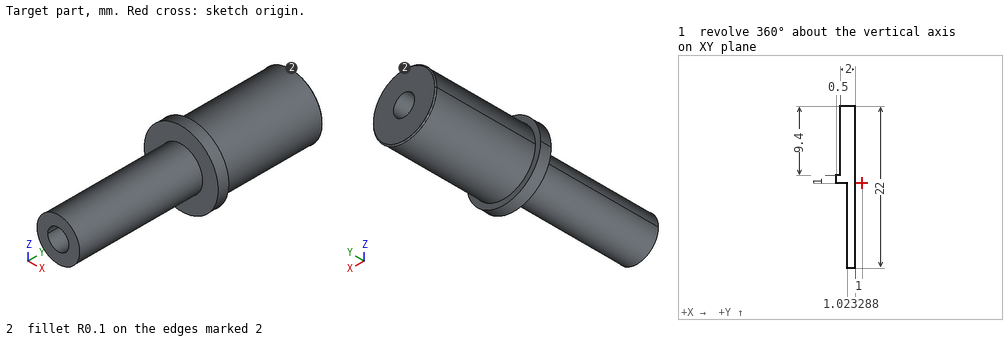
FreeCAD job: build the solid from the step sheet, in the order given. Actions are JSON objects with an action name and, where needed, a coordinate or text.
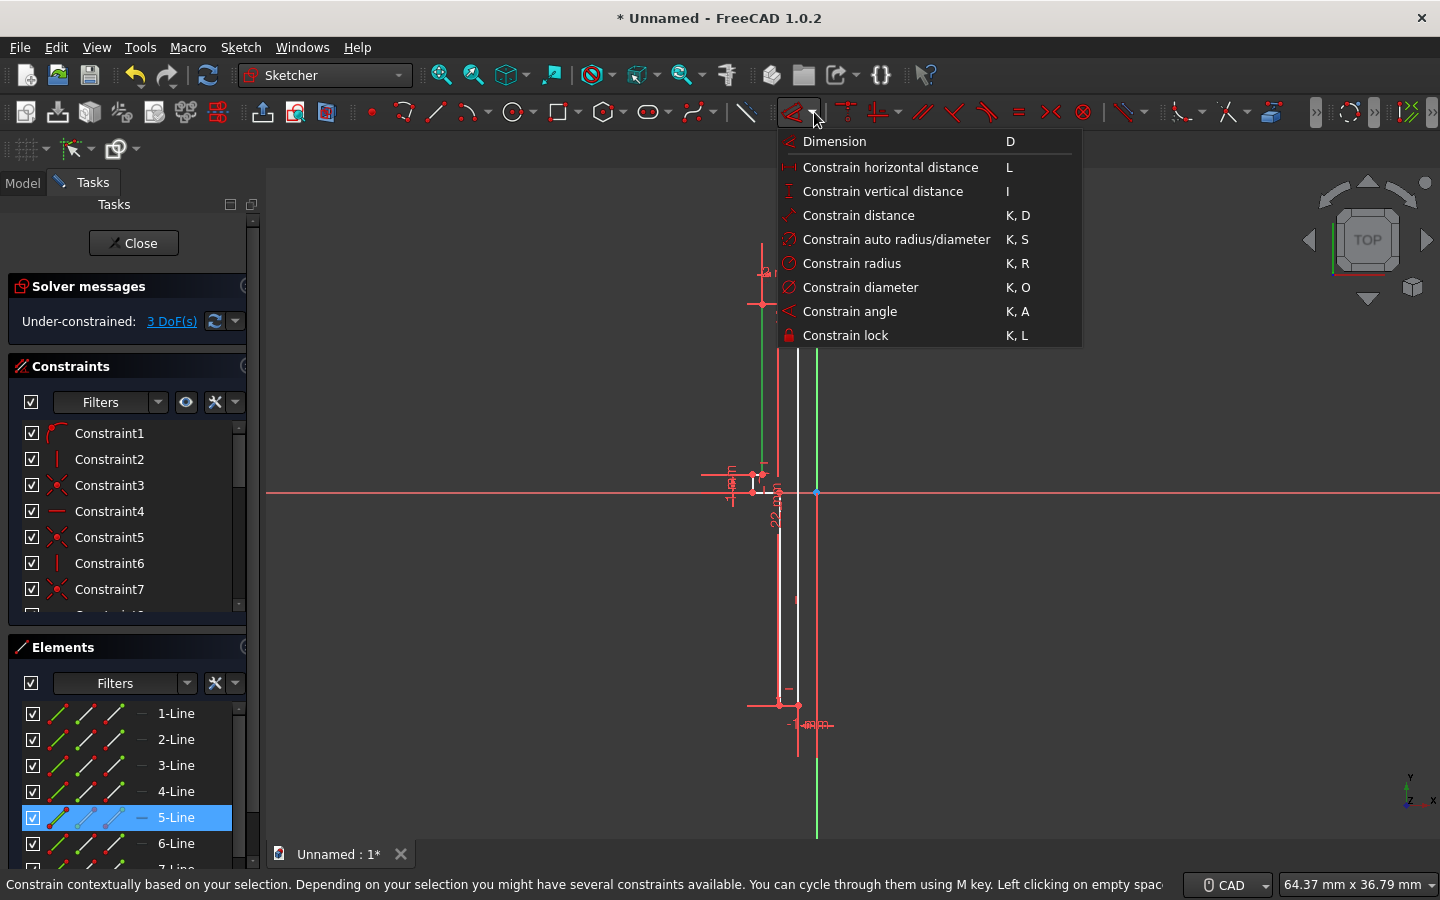
{"action": "left_click", "coordinate": [930, 191]}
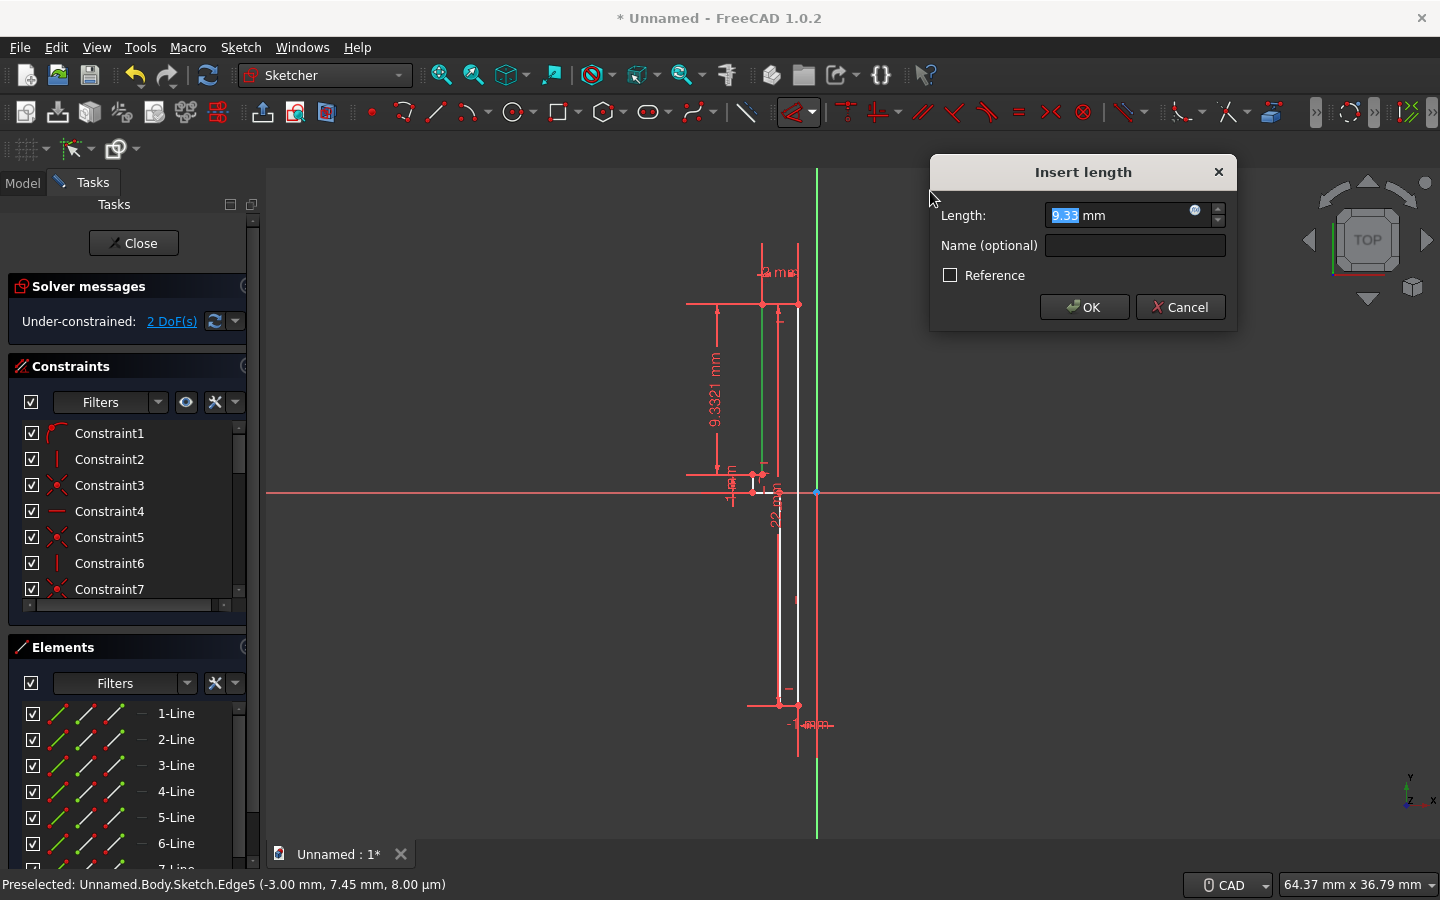
{"action": "type", "text": "9.4"}
{"action": "key", "text": "Return"}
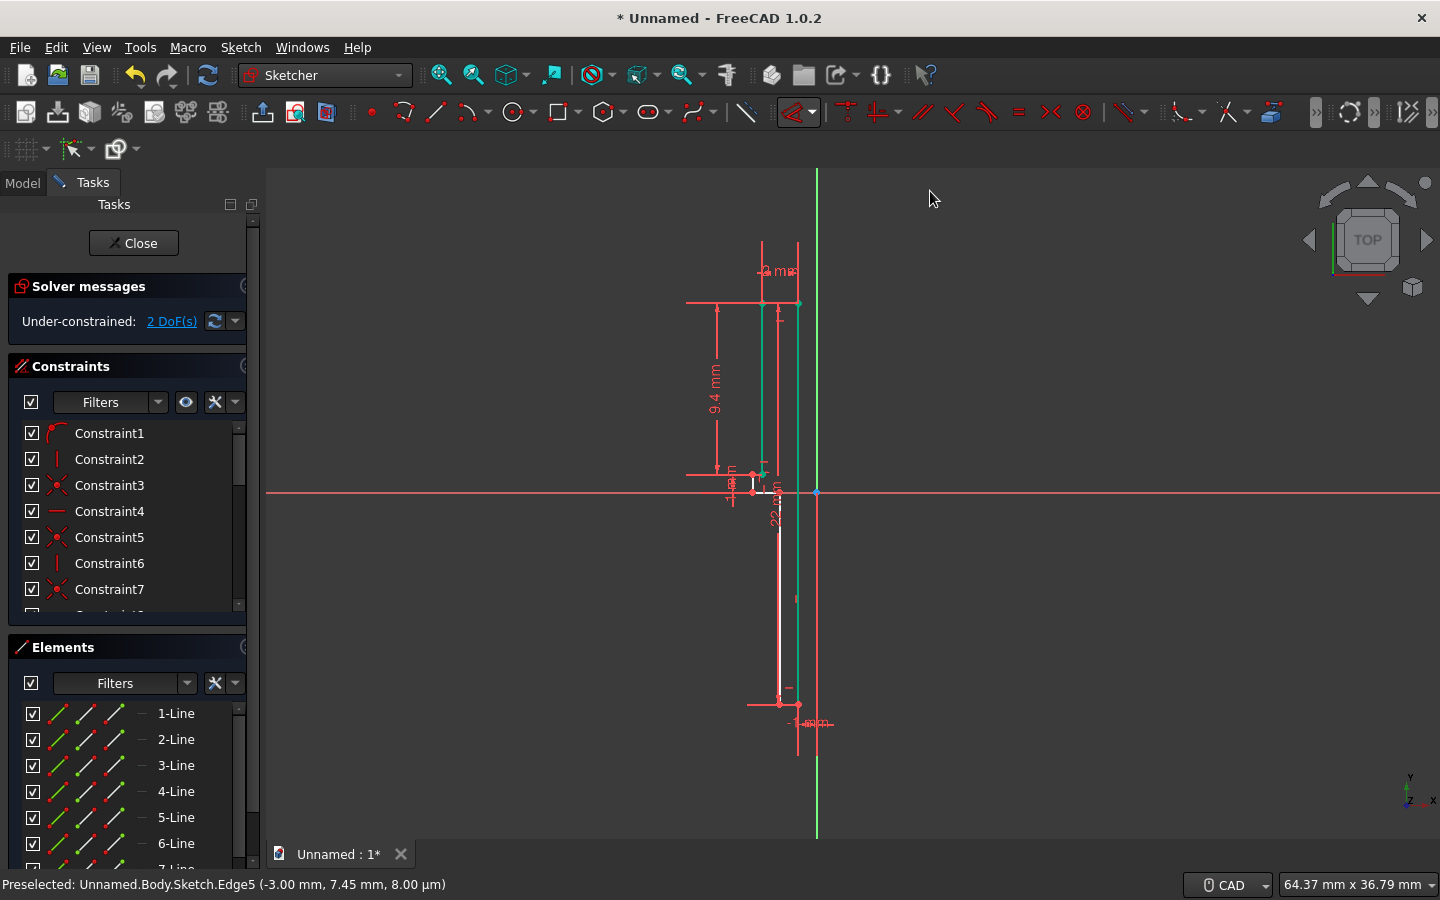
{"action": "scroll", "coordinate": [757, 475], "scroll_direction": "up", "scroll_amount": 8}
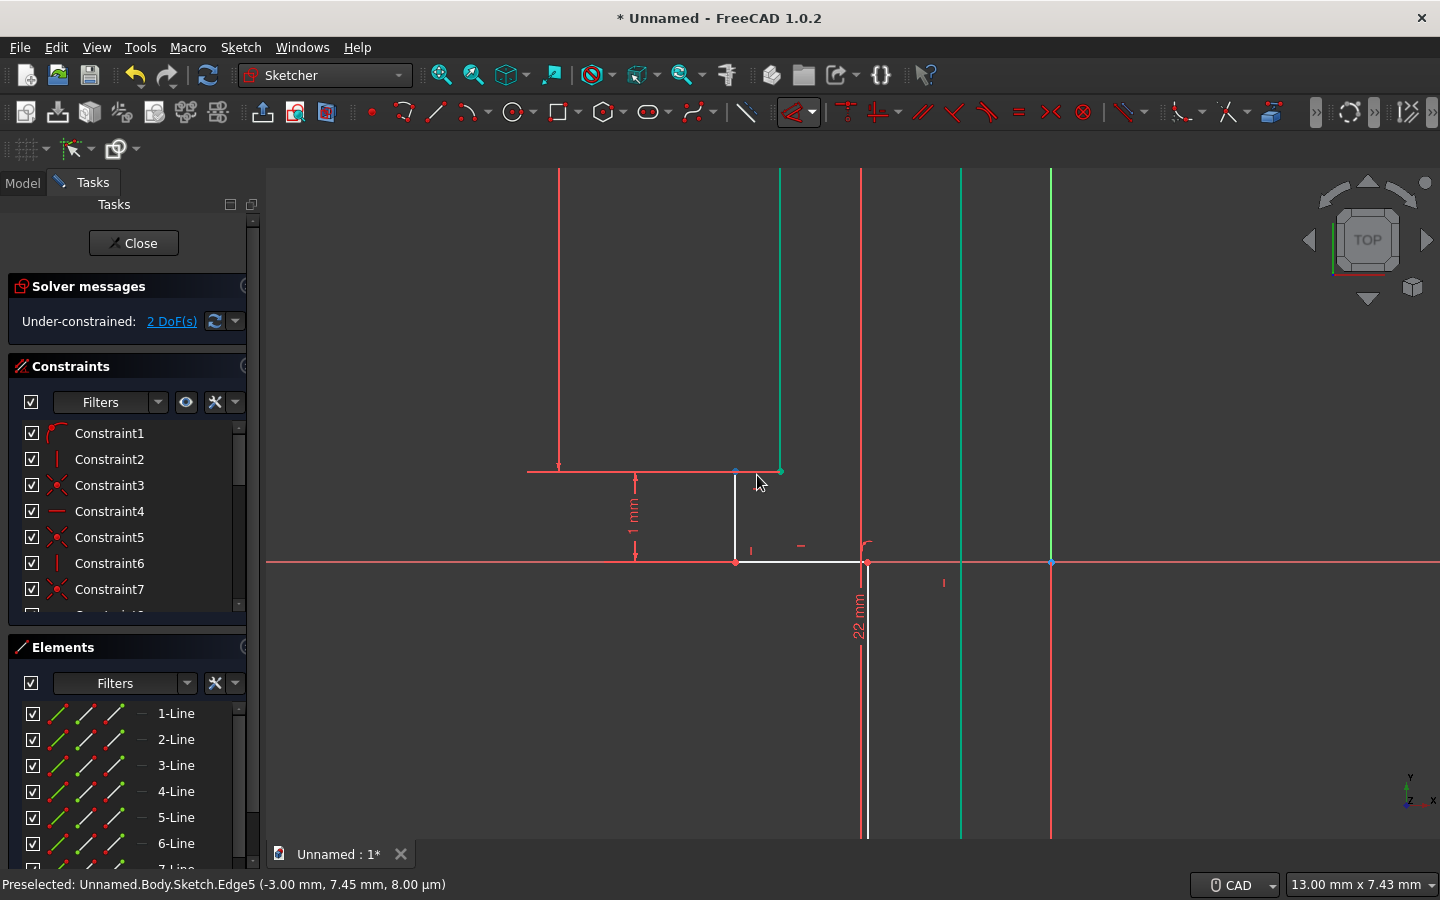
{"action": "left_click", "coordinate": [758, 472]}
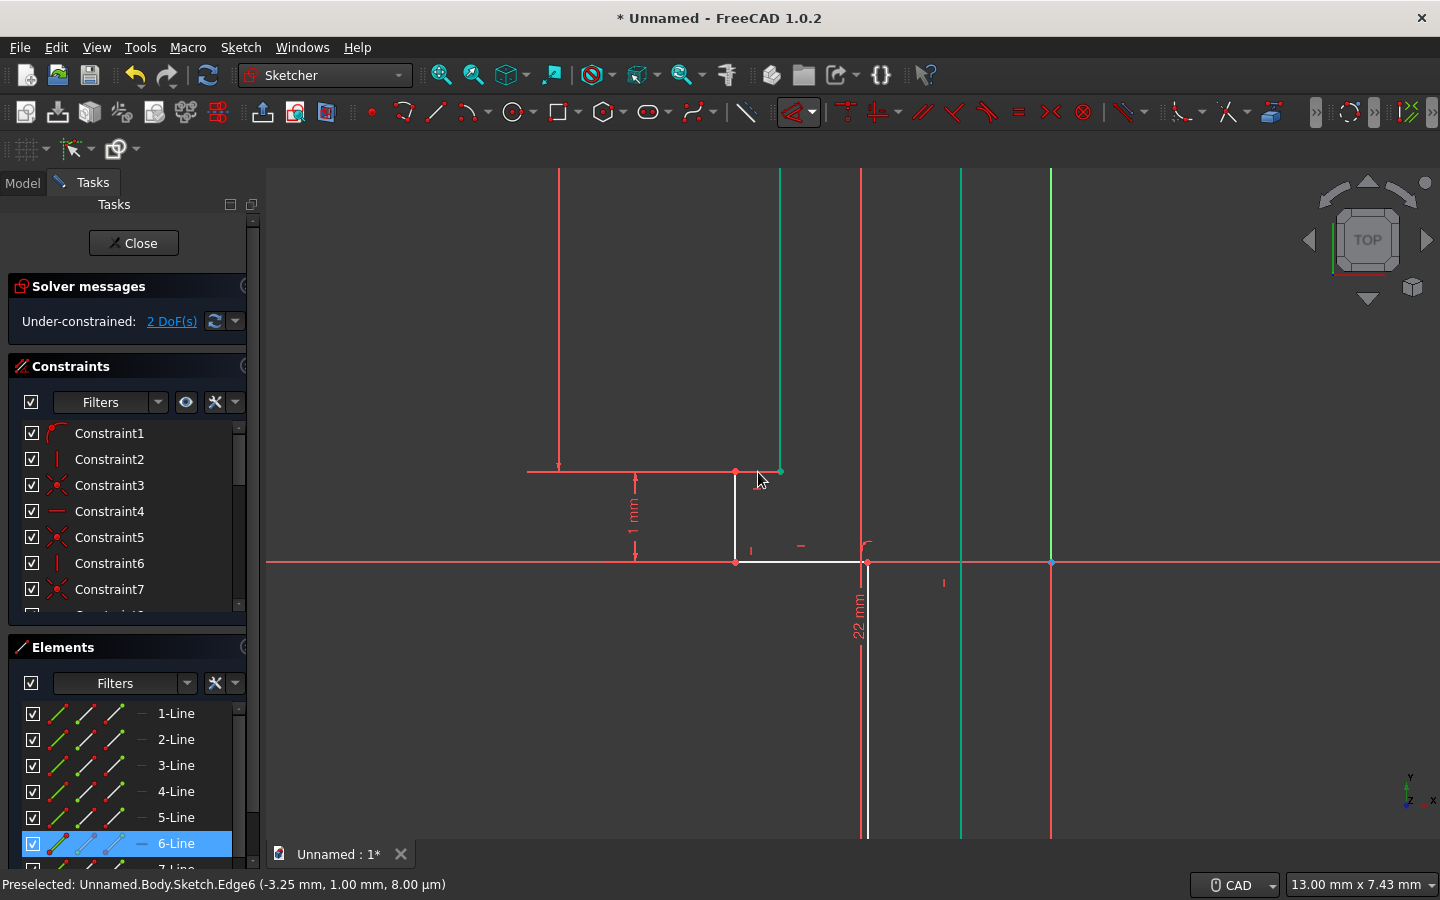
{"action": "left_click", "coordinate": [814, 112]}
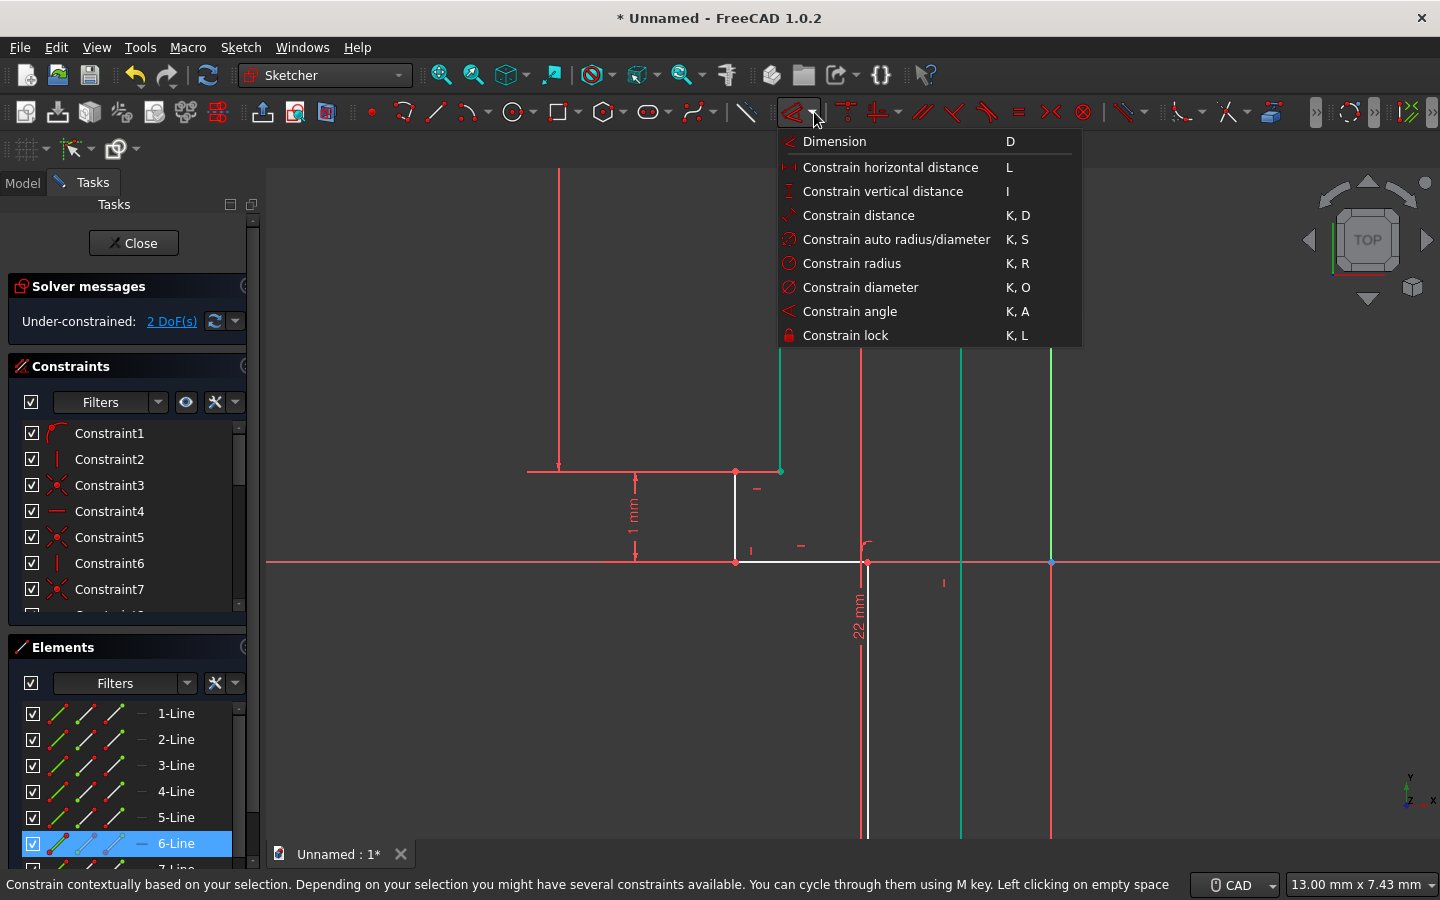
{"action": "left_click", "coordinate": [930, 167]}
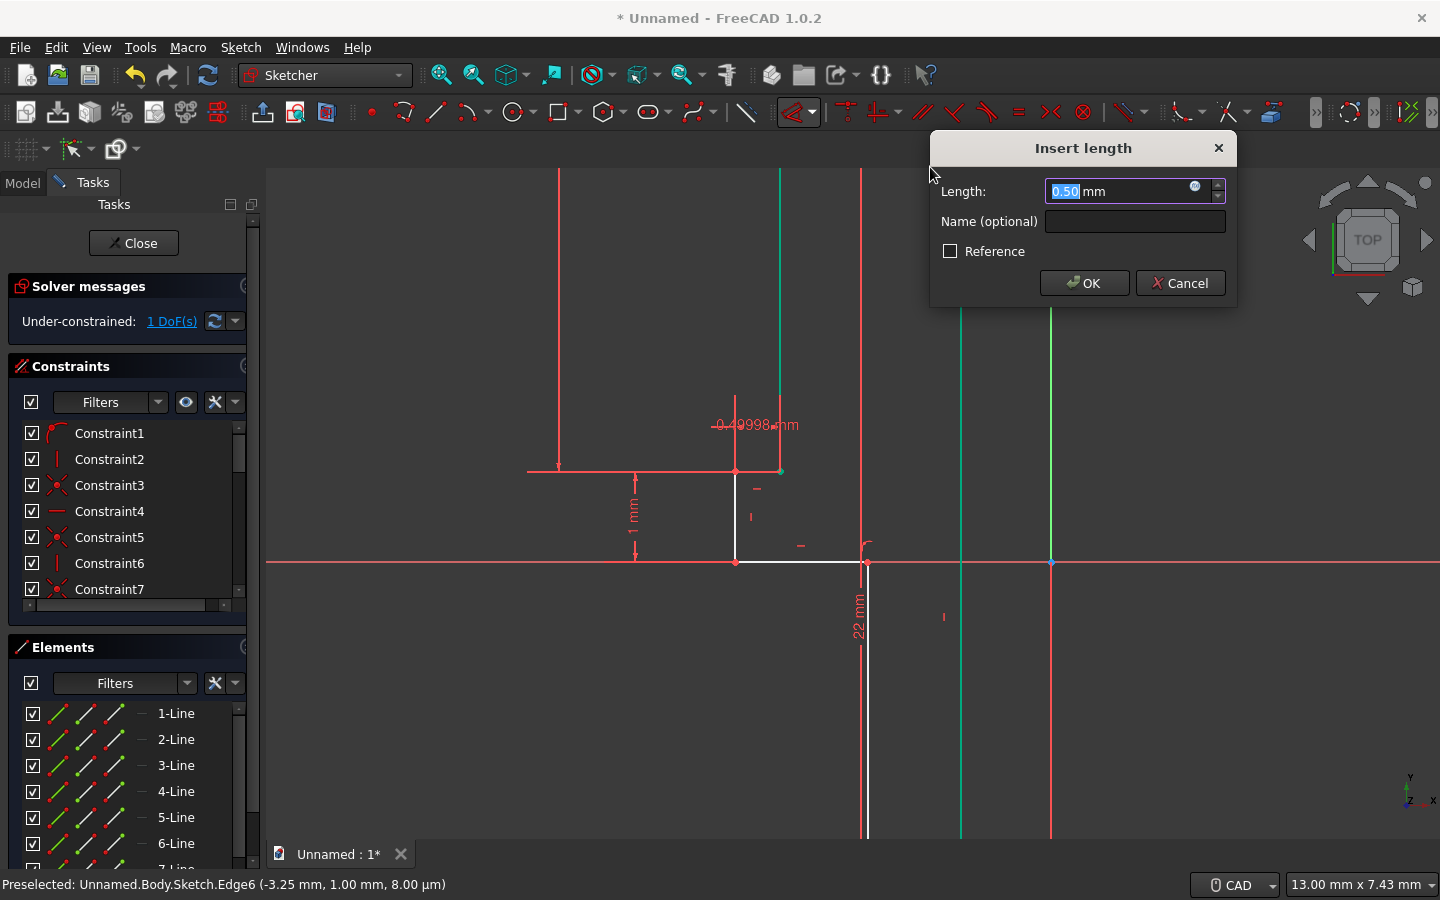
{"action": "type", "text": "0.5"}
{"action": "key", "text": "Return"}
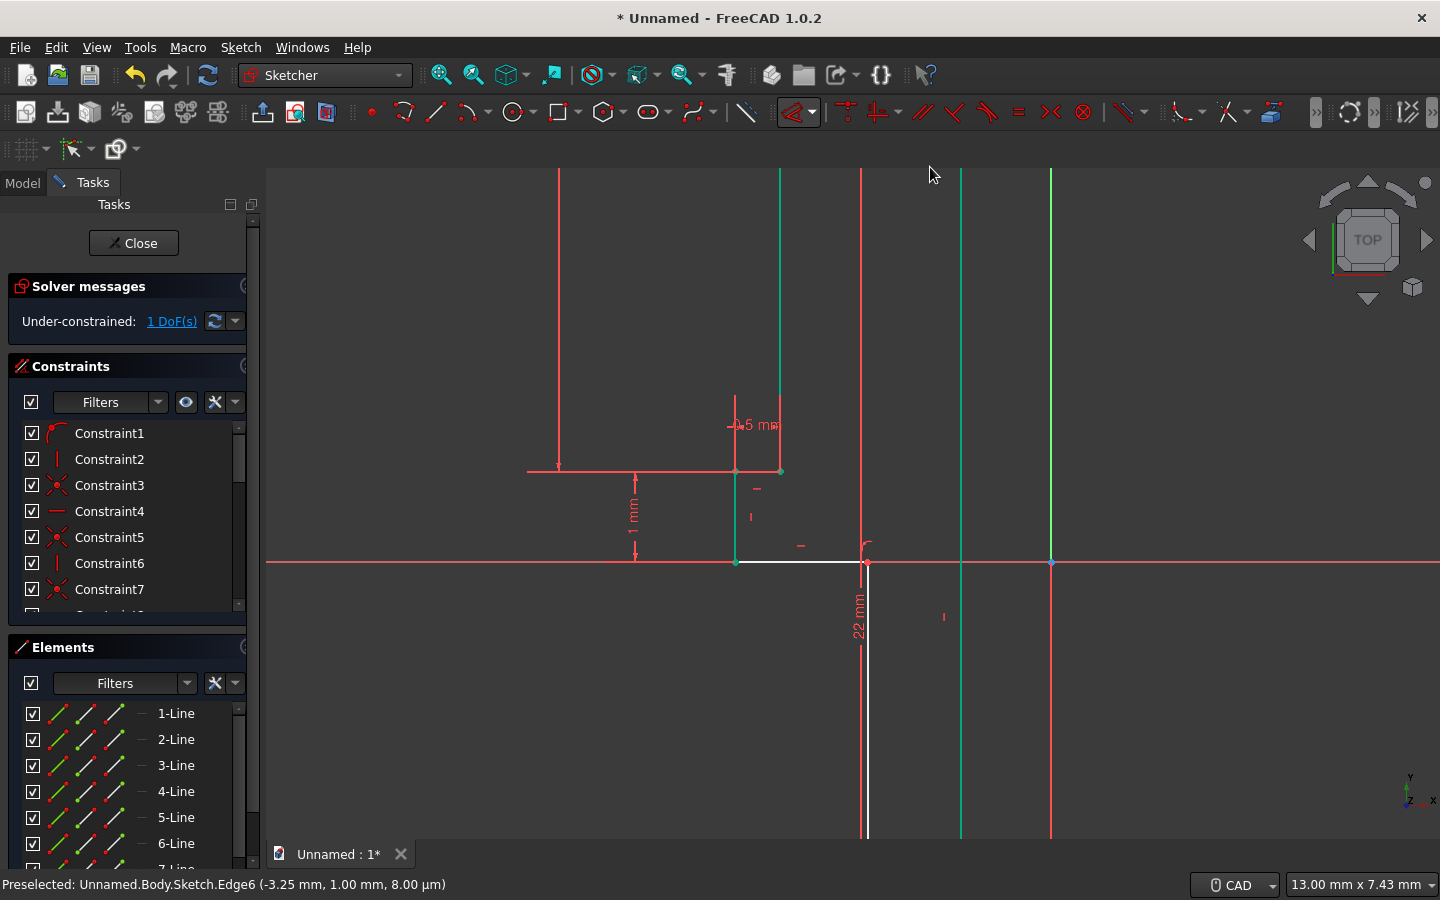
{"action": "scroll", "coordinate": [757, 475], "scroll_direction": "down", "scroll_amount": 8}